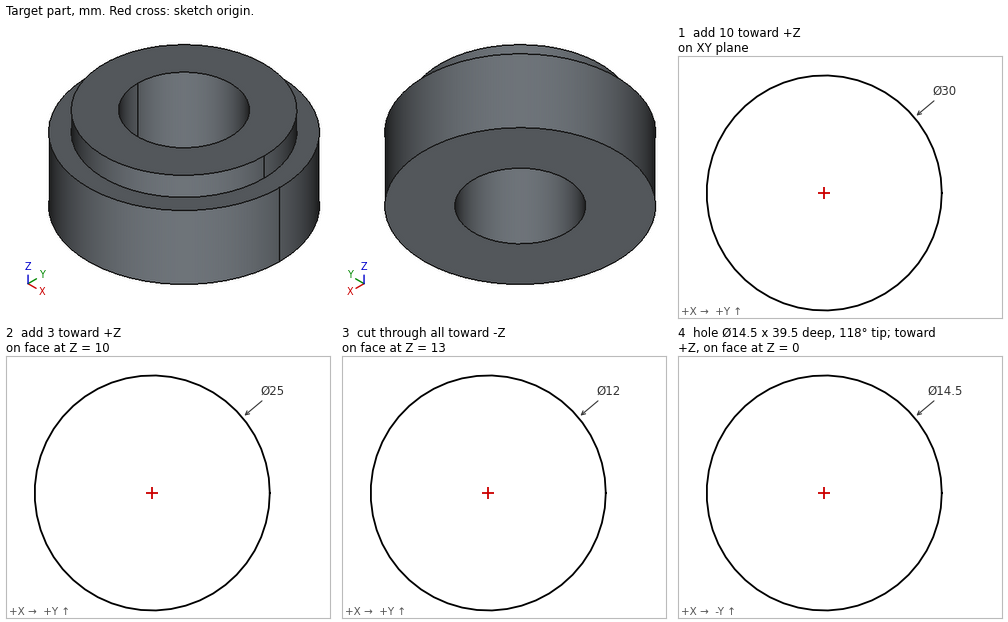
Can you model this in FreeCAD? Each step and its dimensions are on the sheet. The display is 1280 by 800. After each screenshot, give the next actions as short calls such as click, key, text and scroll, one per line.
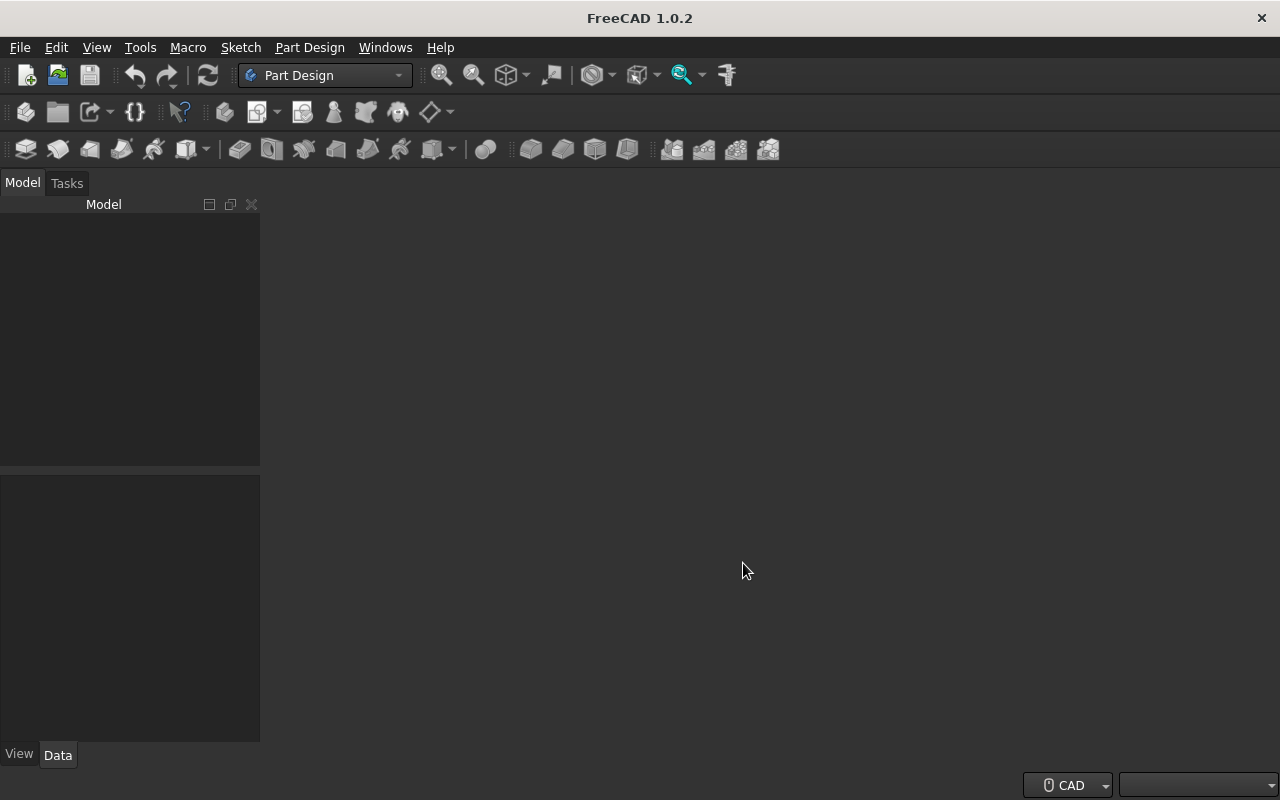
click(26, 76)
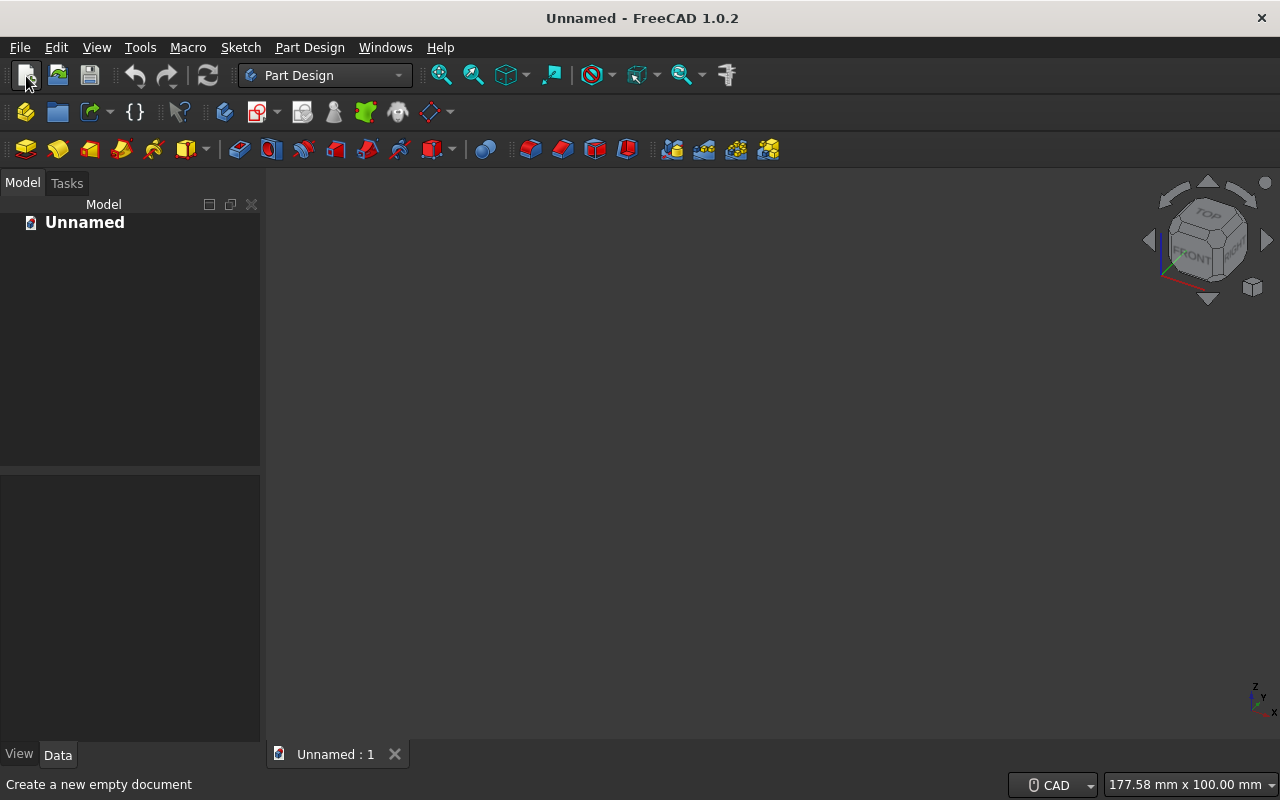
click(258, 112)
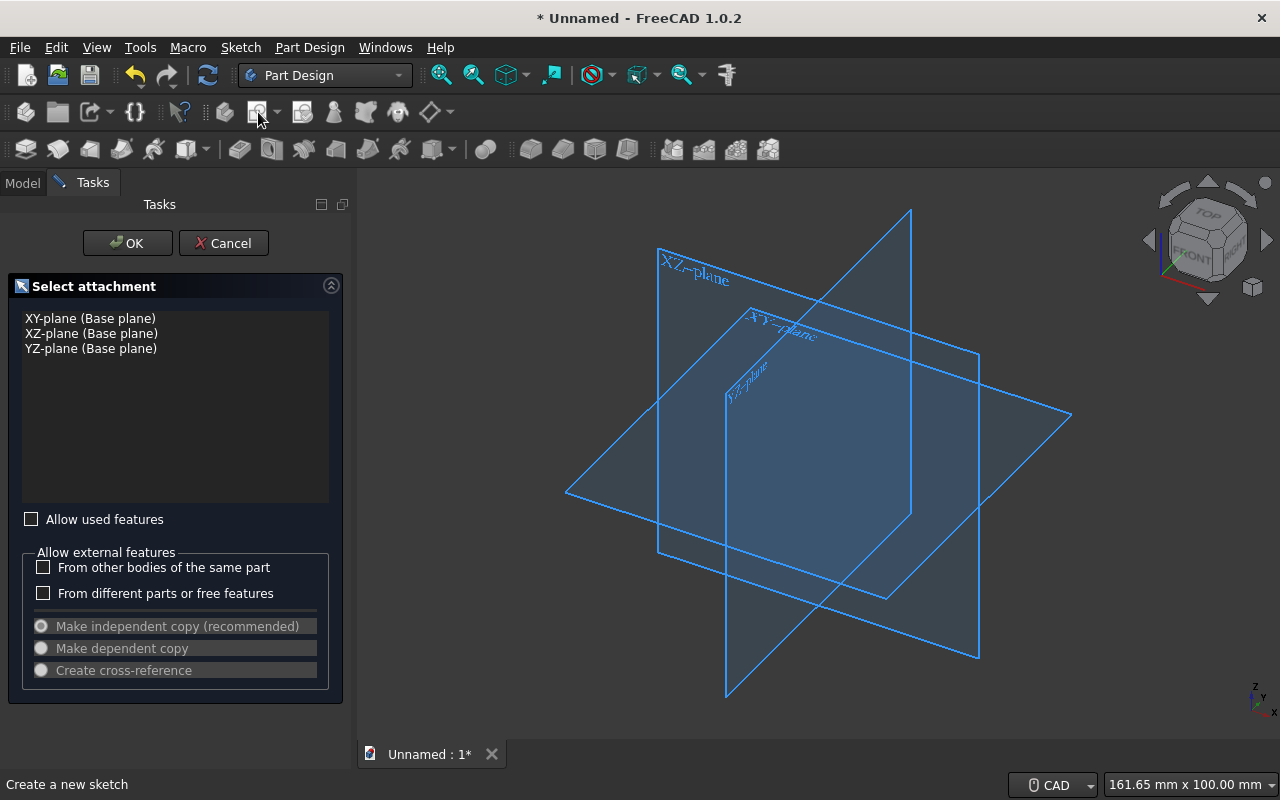
click(82, 318)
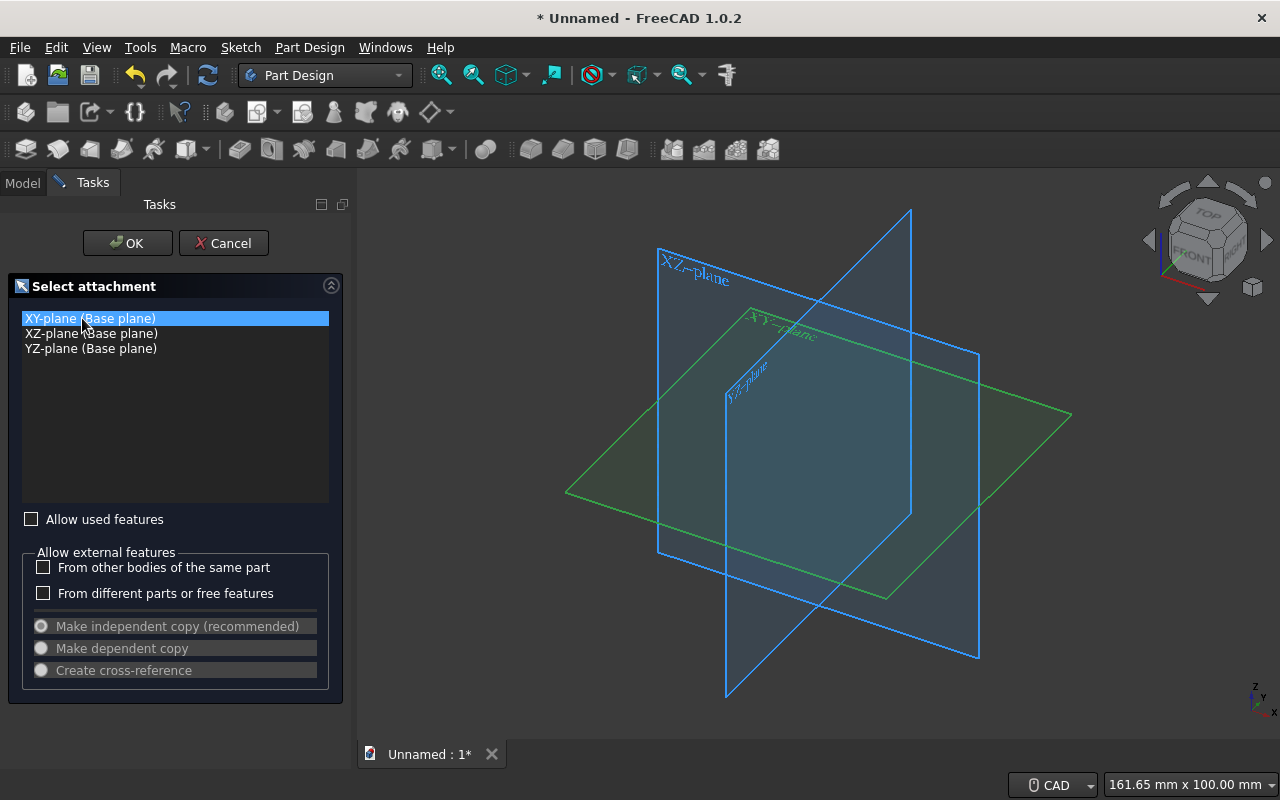
click(128, 243)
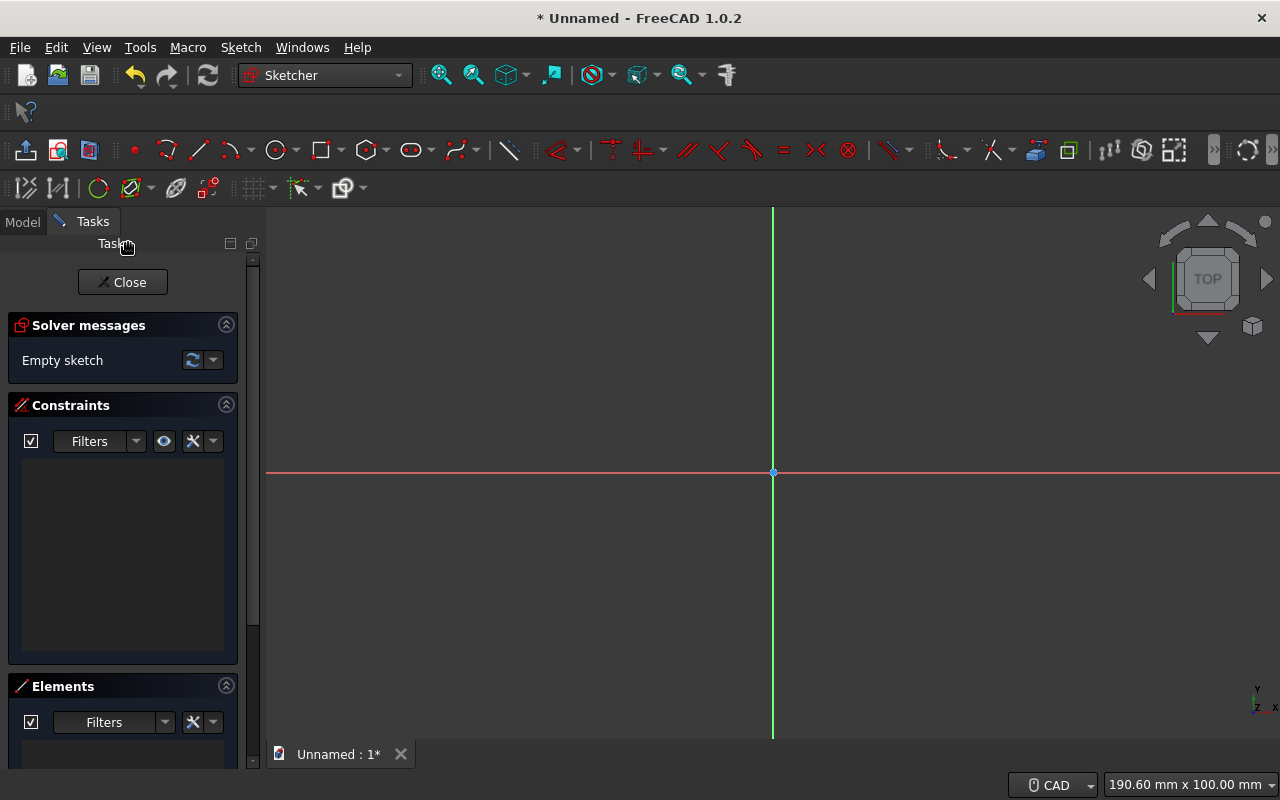
scroll(829, 473, up, 4)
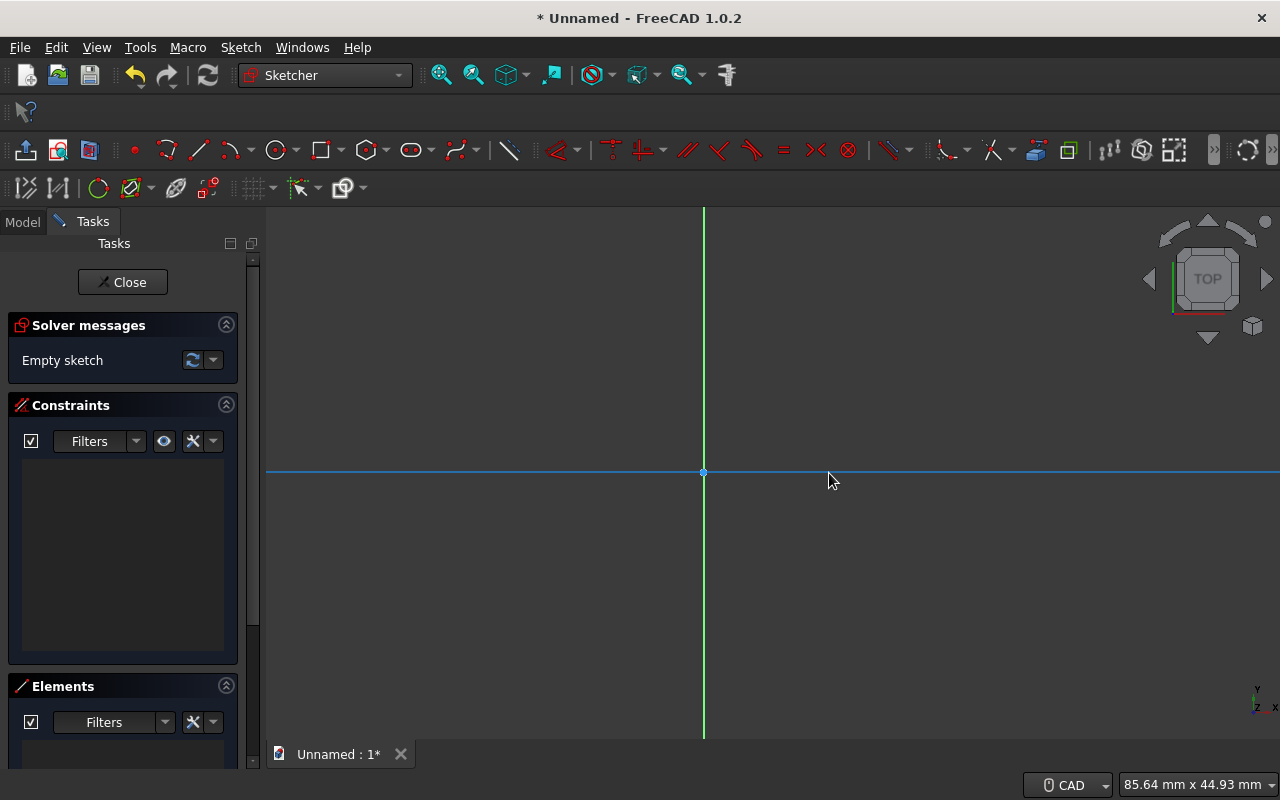
click(276, 150)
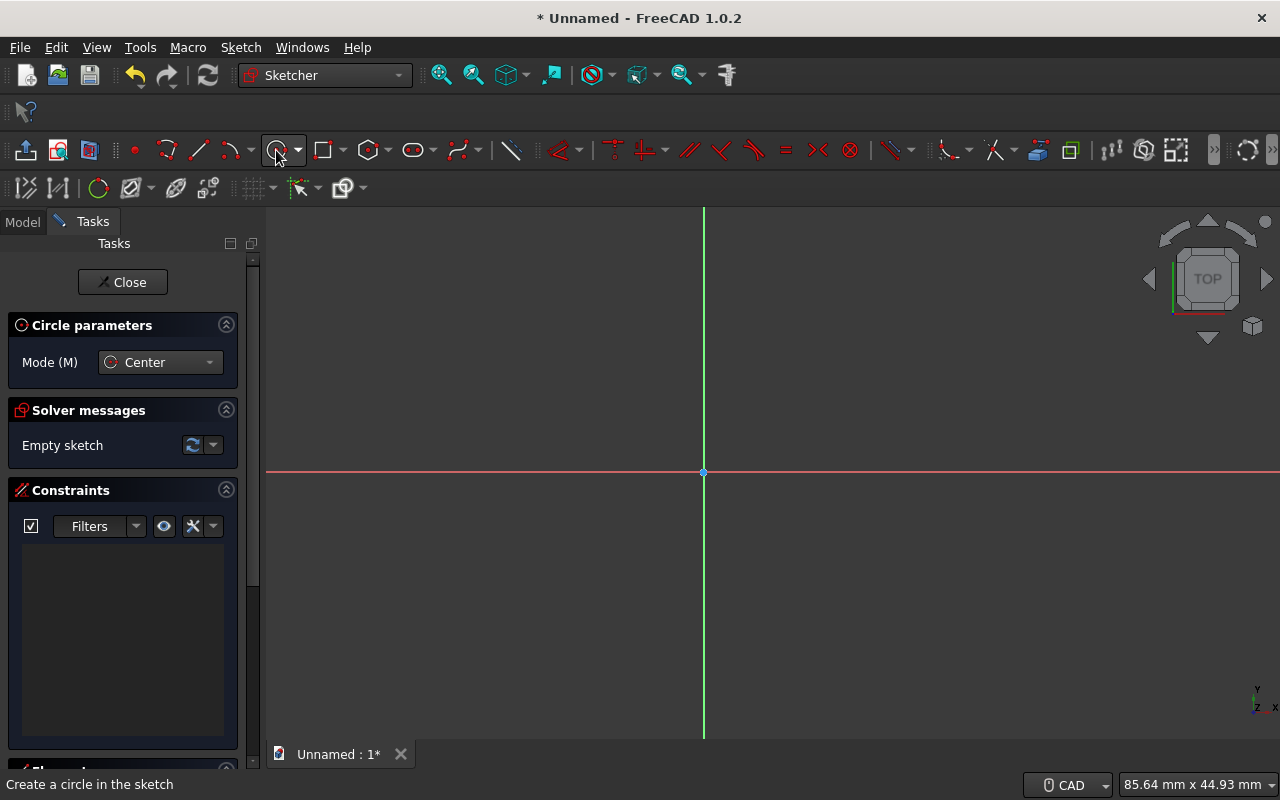
click(704, 472)
click(829, 347)
key(Escape)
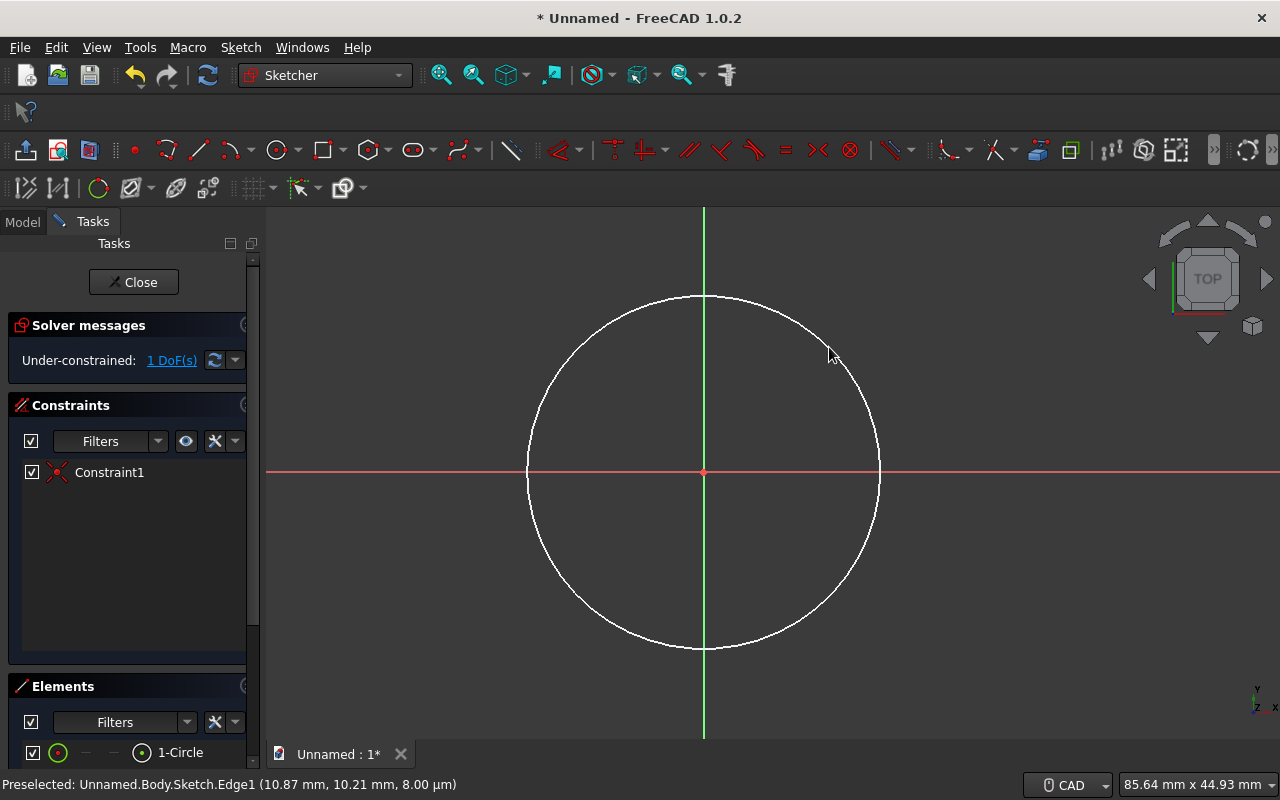
click(558, 150)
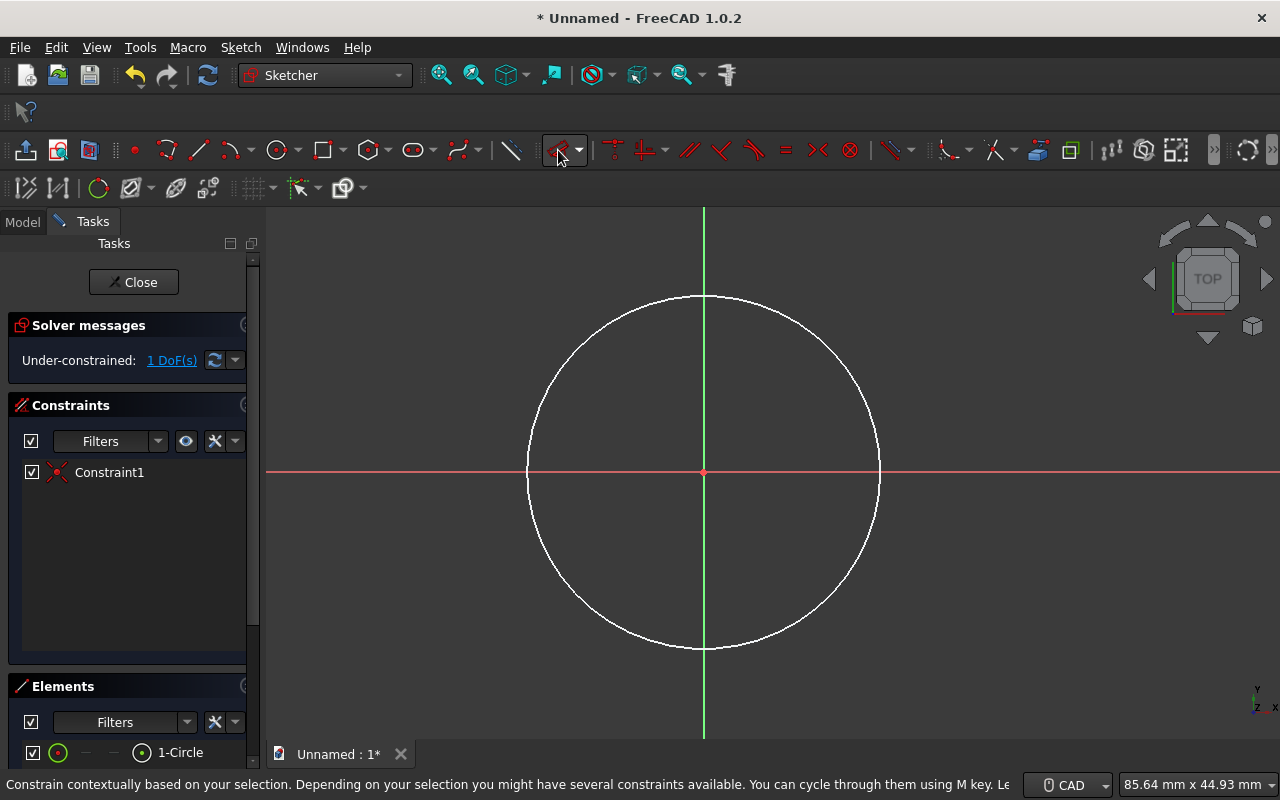
click(828, 347)
click(851, 324)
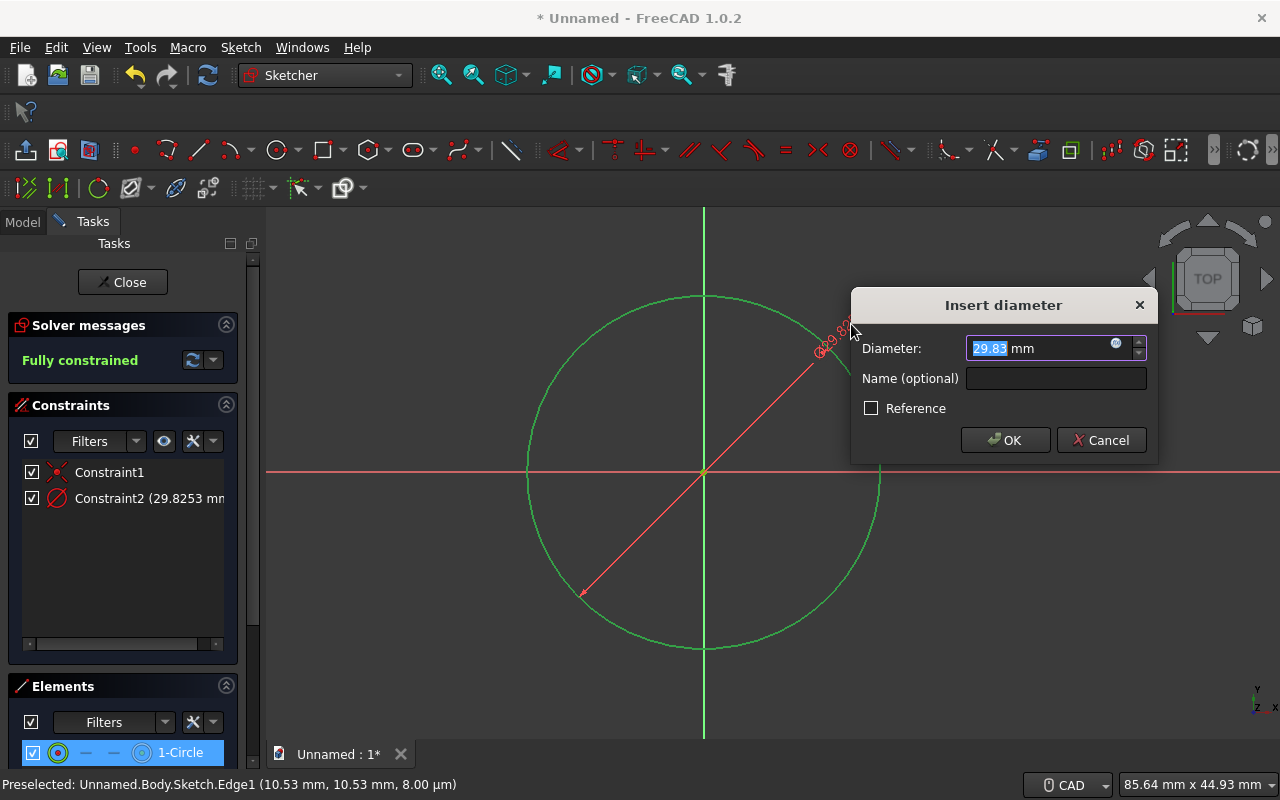
text(30)
key(Return)
key(Escape)